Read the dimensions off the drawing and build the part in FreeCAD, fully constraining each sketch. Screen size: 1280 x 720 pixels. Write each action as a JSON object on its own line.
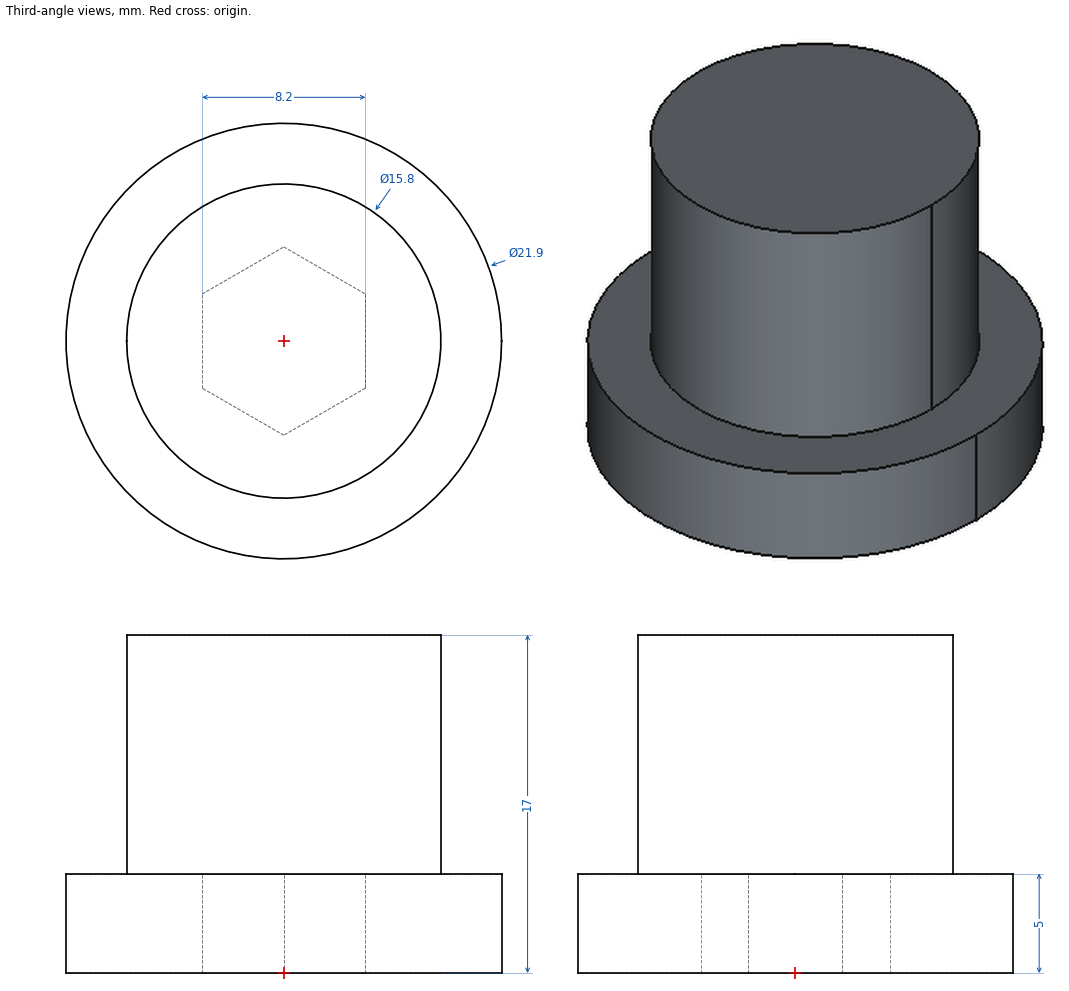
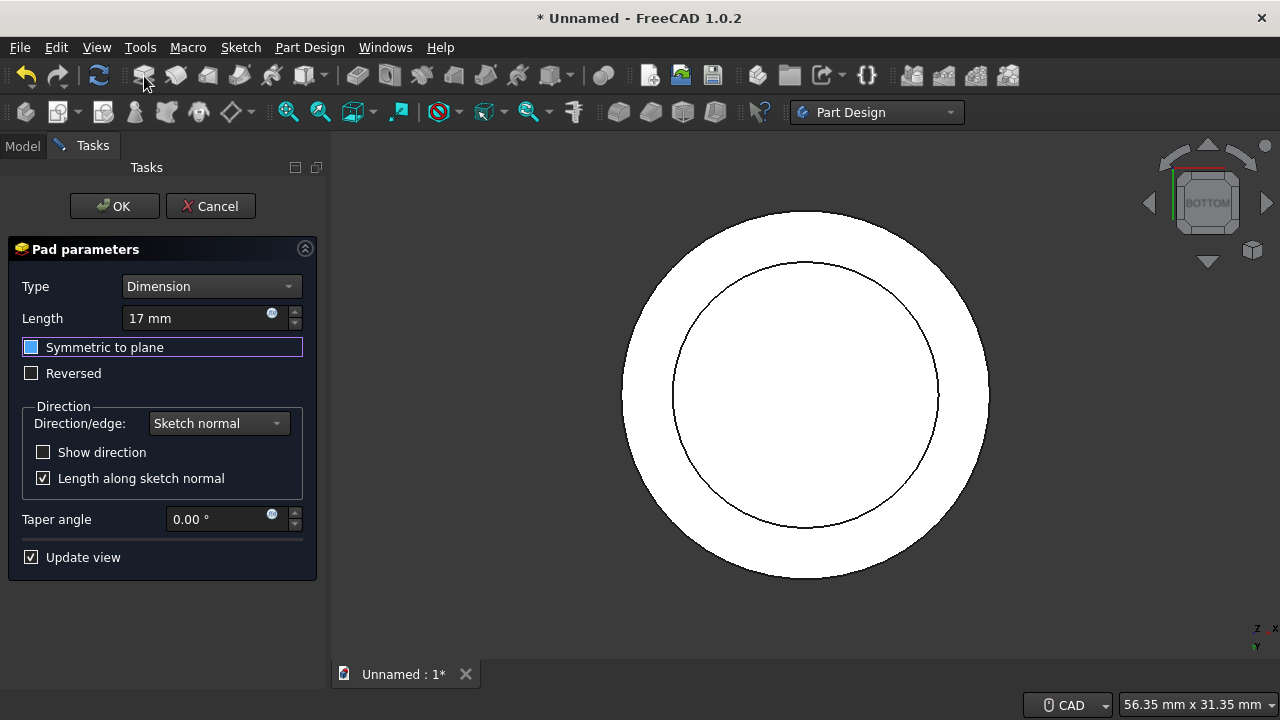
{"action": "left_click", "coordinate": [30, 373]}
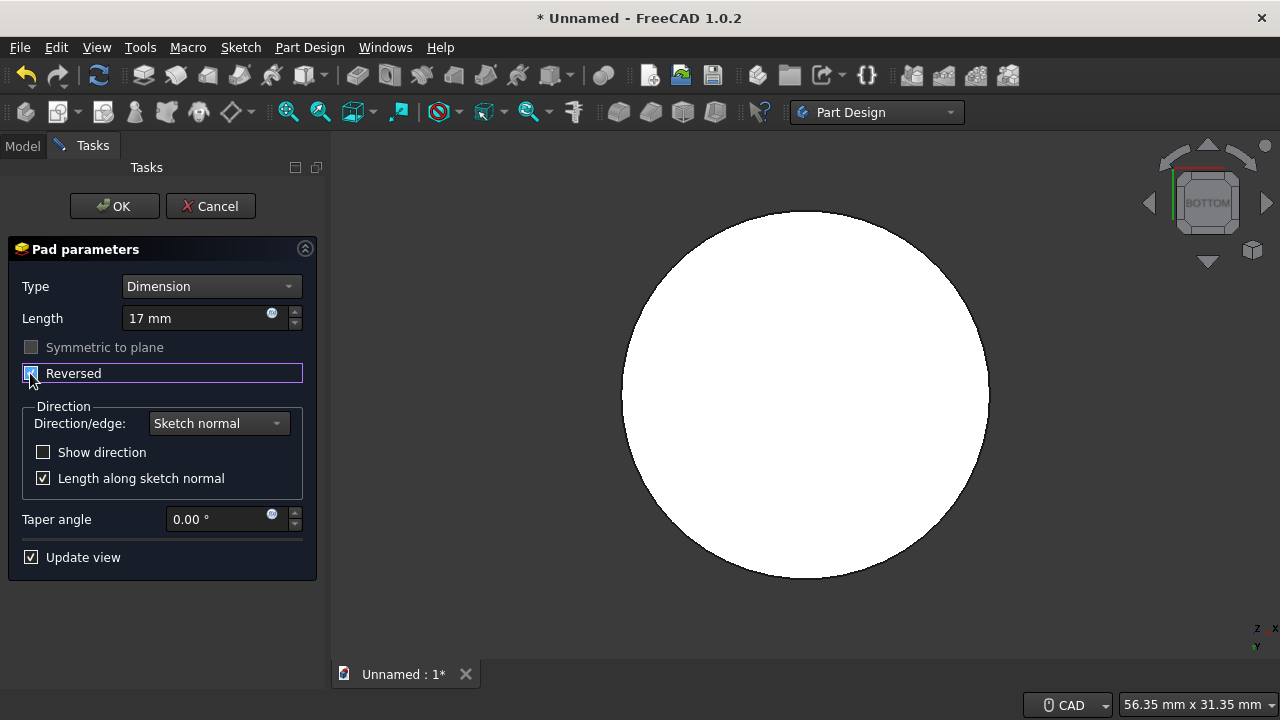
{"action": "left_click", "coordinate": [115, 206]}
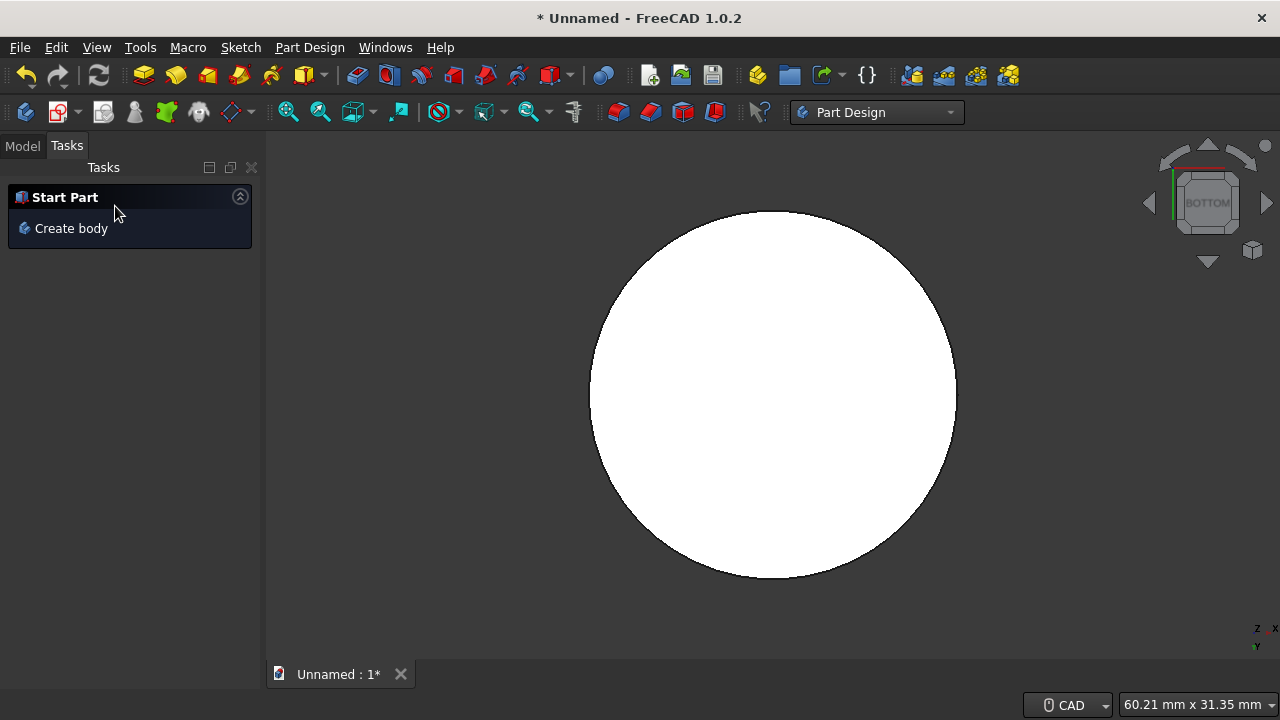
{"action": "left_click", "coordinate": [58, 112]}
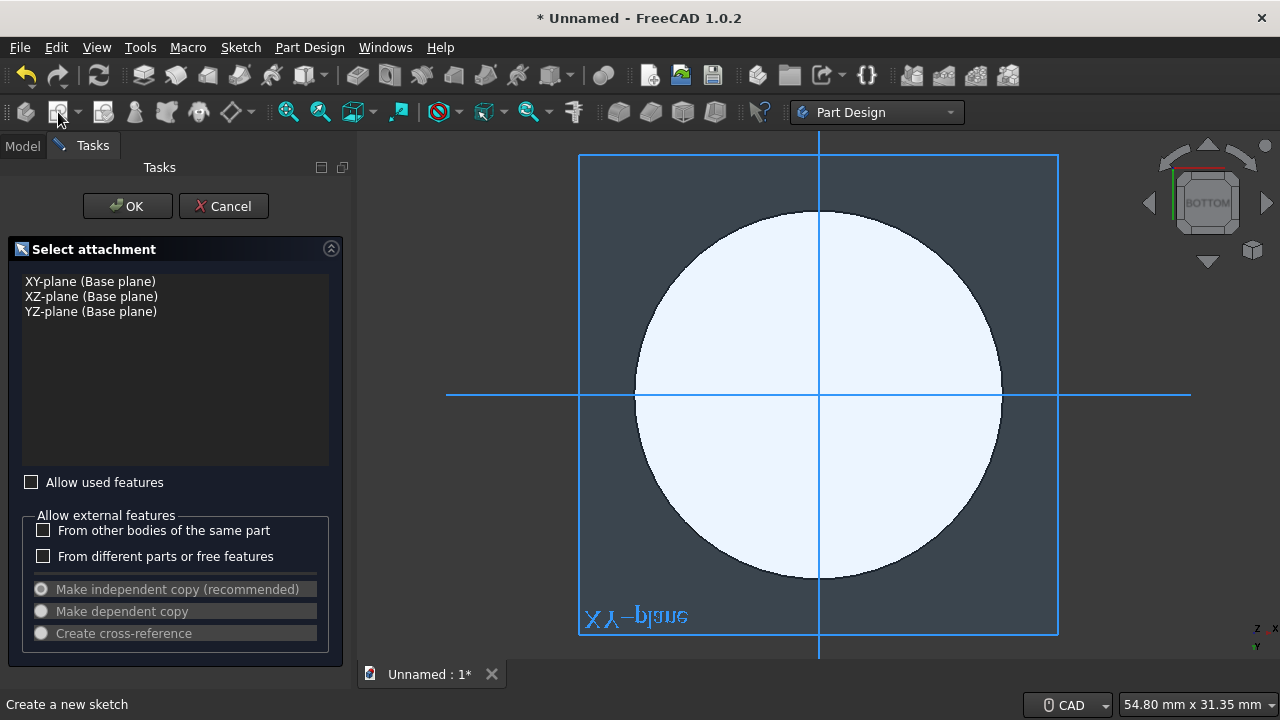
{"action": "left_click", "coordinate": [82, 282]}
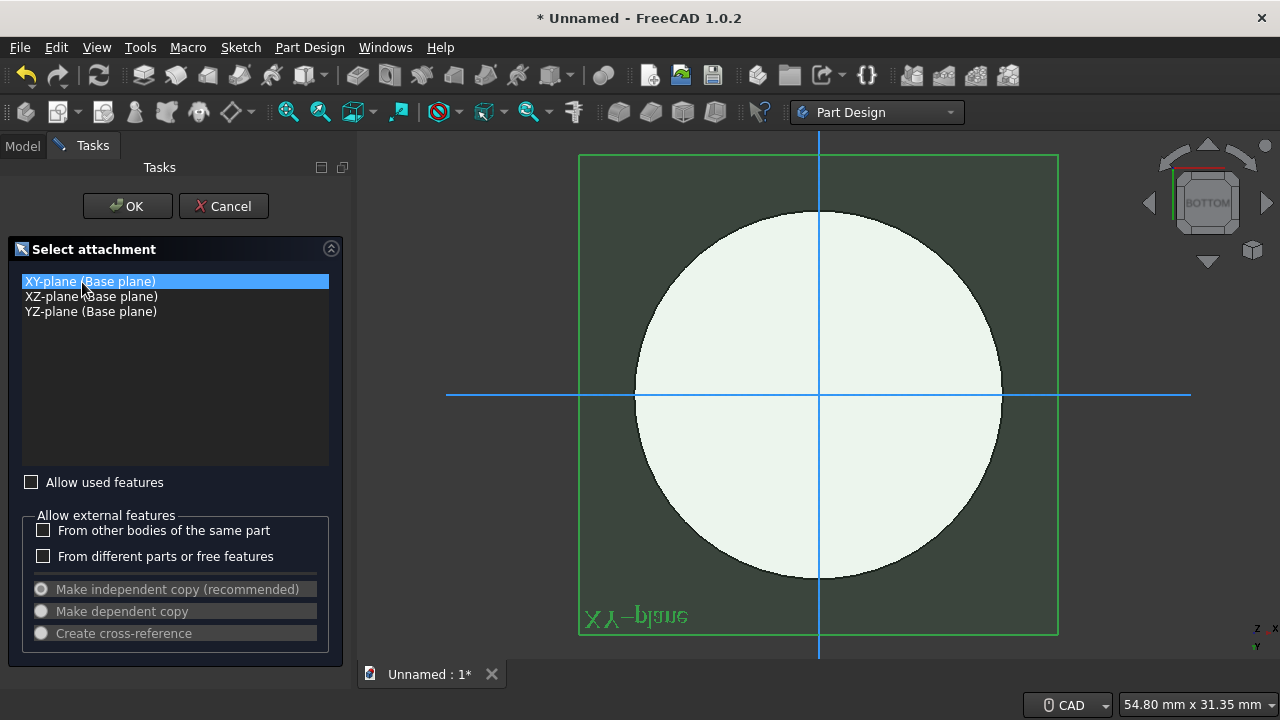
{"action": "left_click", "coordinate": [128, 206]}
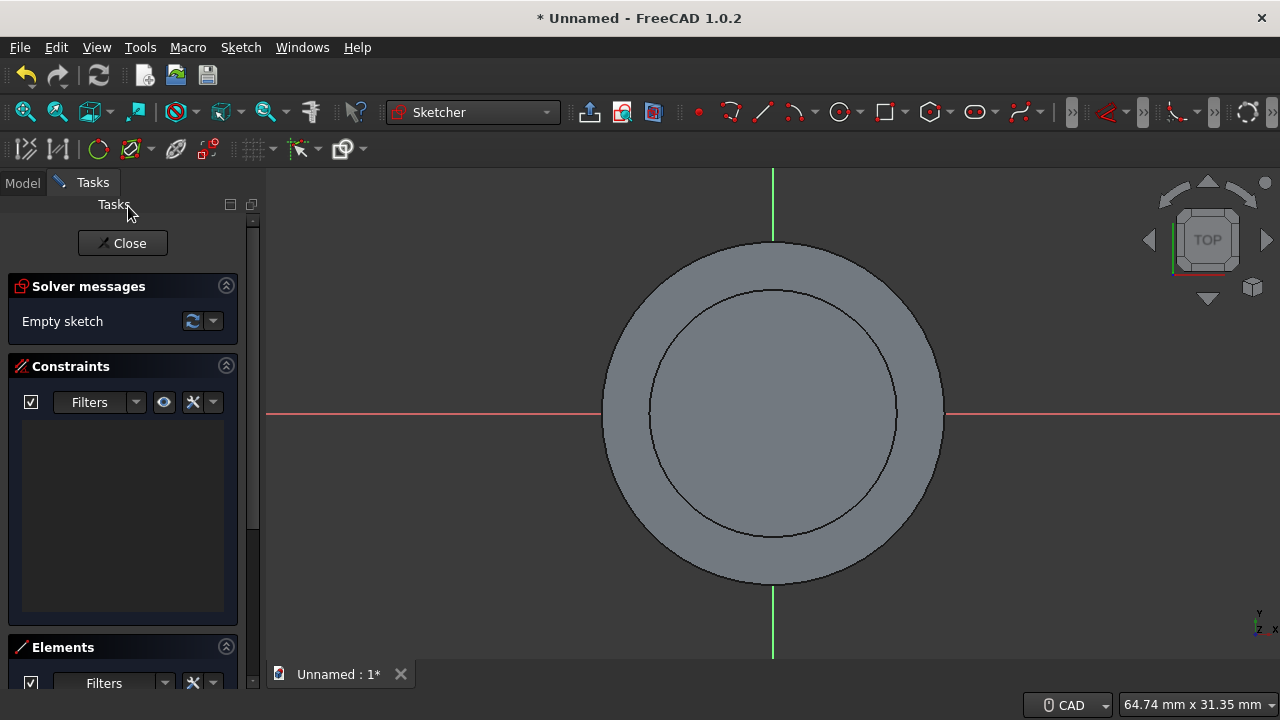
{"action": "key", "text": "q s"}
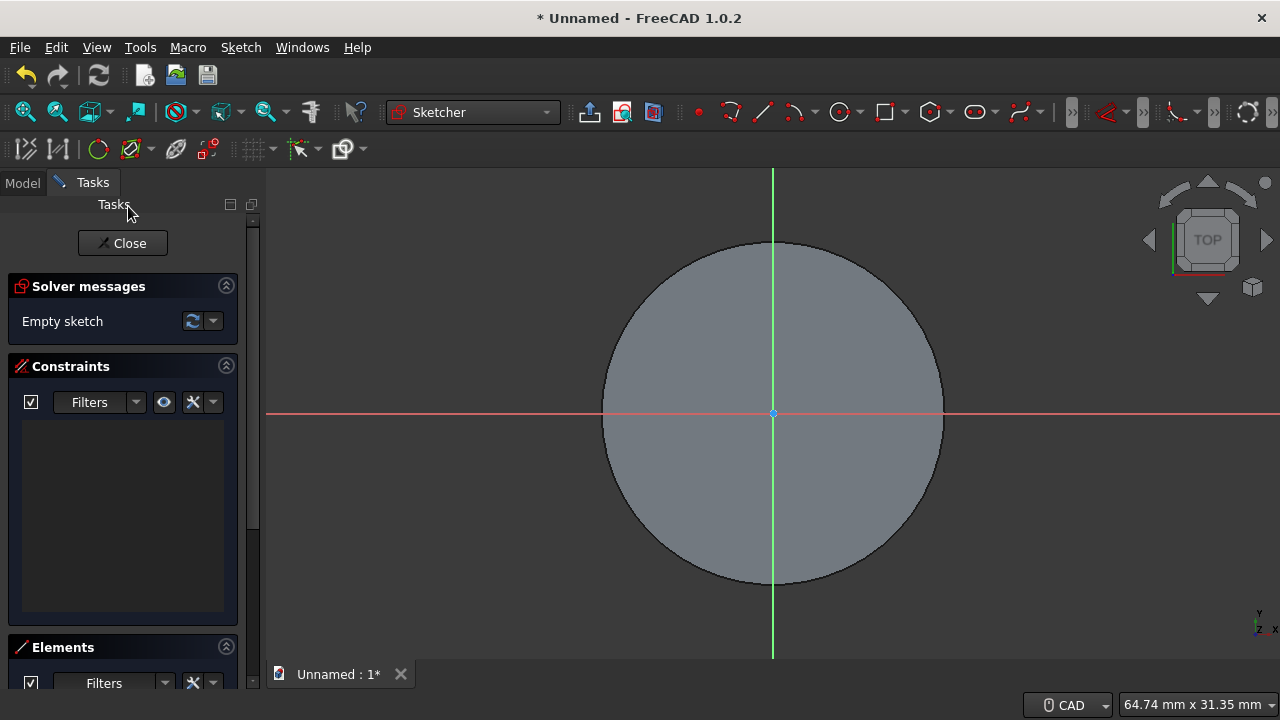
{"action": "scroll", "coordinate": [829, 413], "scroll_direction": "up", "scroll_amount": 4}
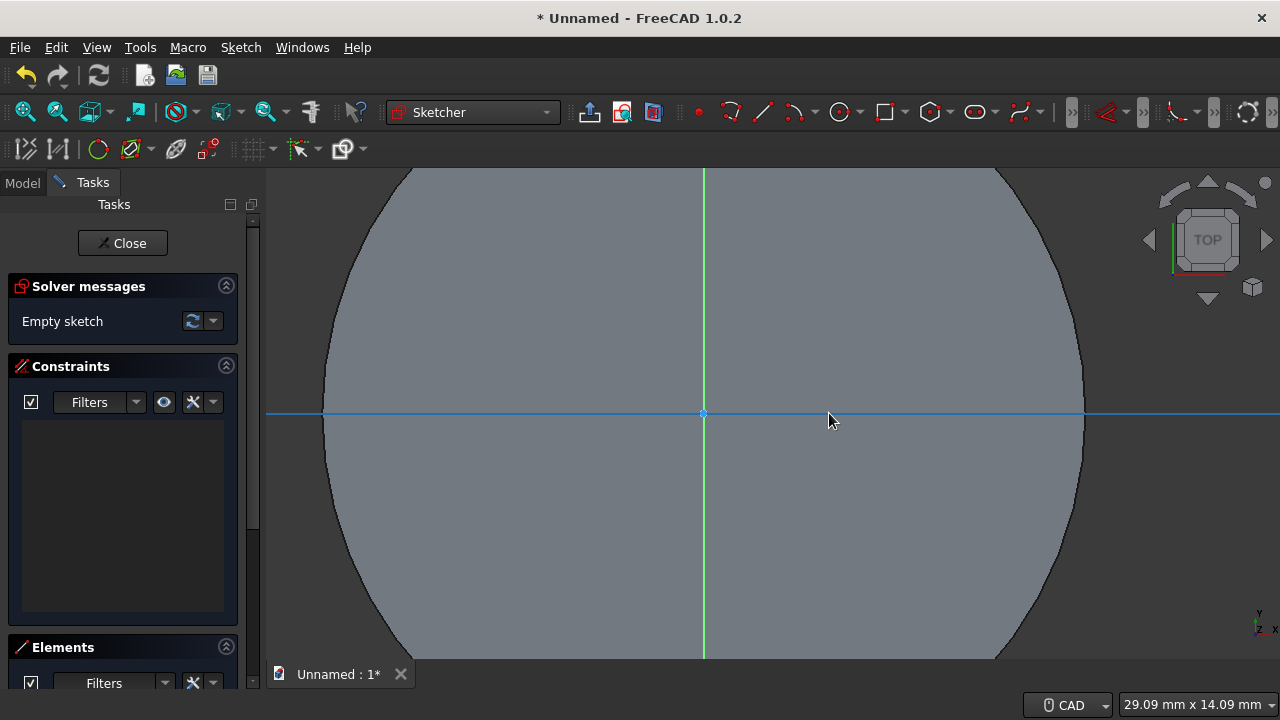
{"action": "key", "text": "g p 6"}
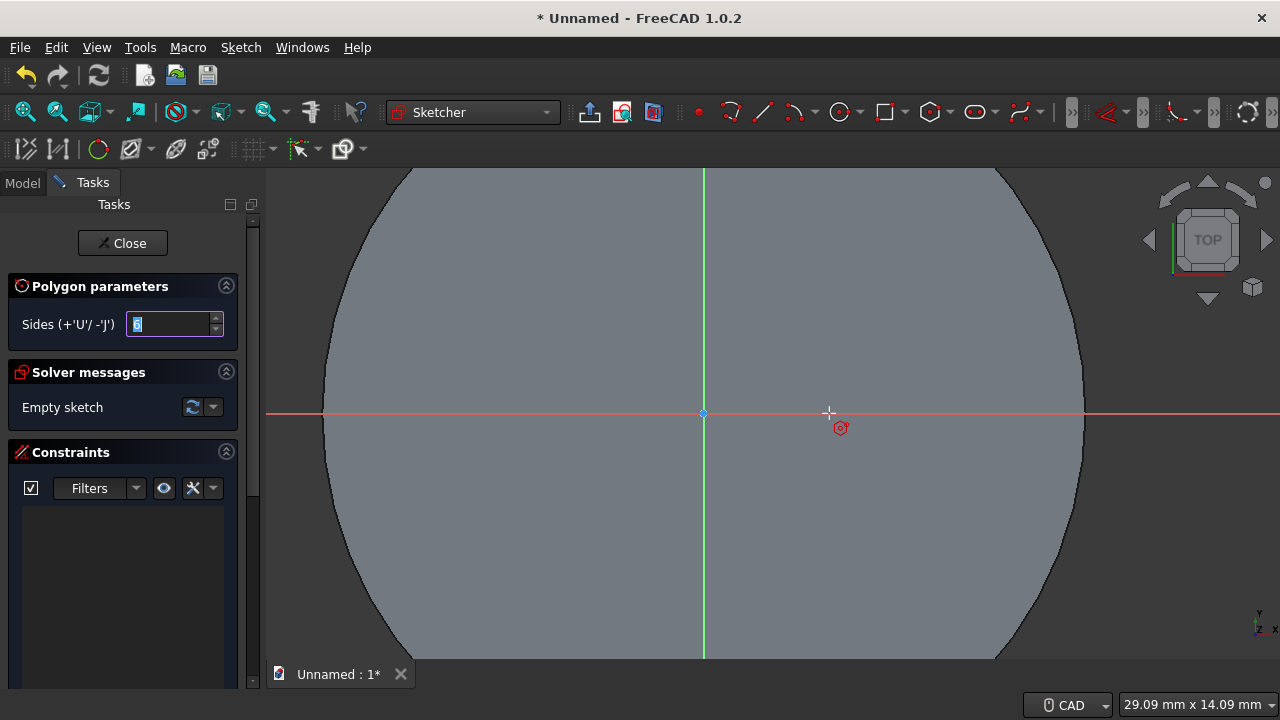
{"action": "left_click", "coordinate": [704, 413]}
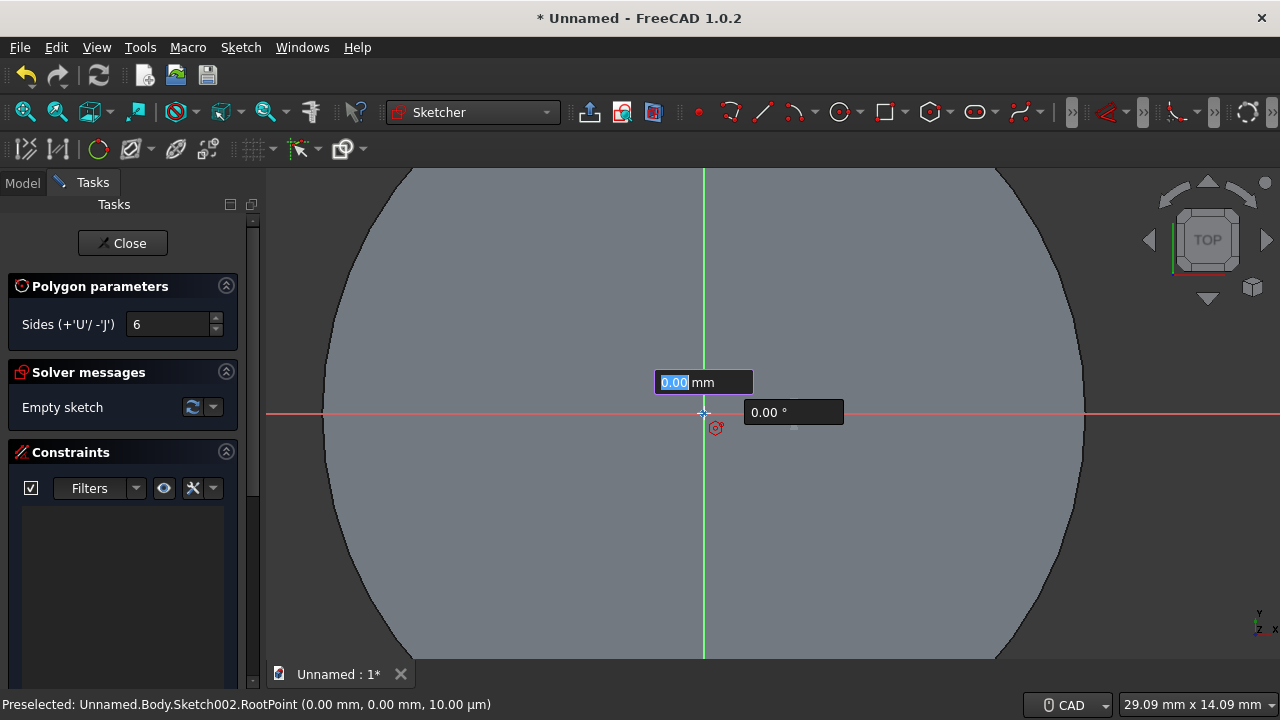
{"action": "left_click", "coordinate": [704, 248]}
{"action": "right_click", "coordinate": [704, 248]}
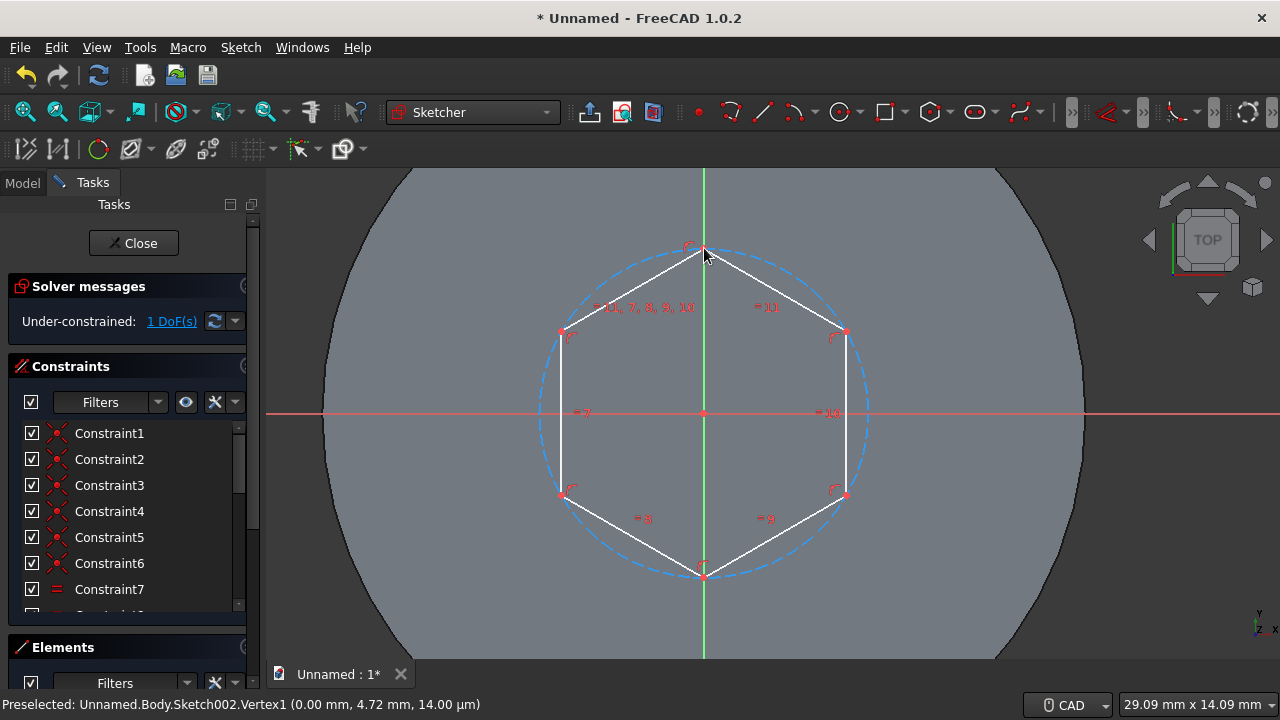
{"action": "left_click", "coordinate": [1106, 112]}